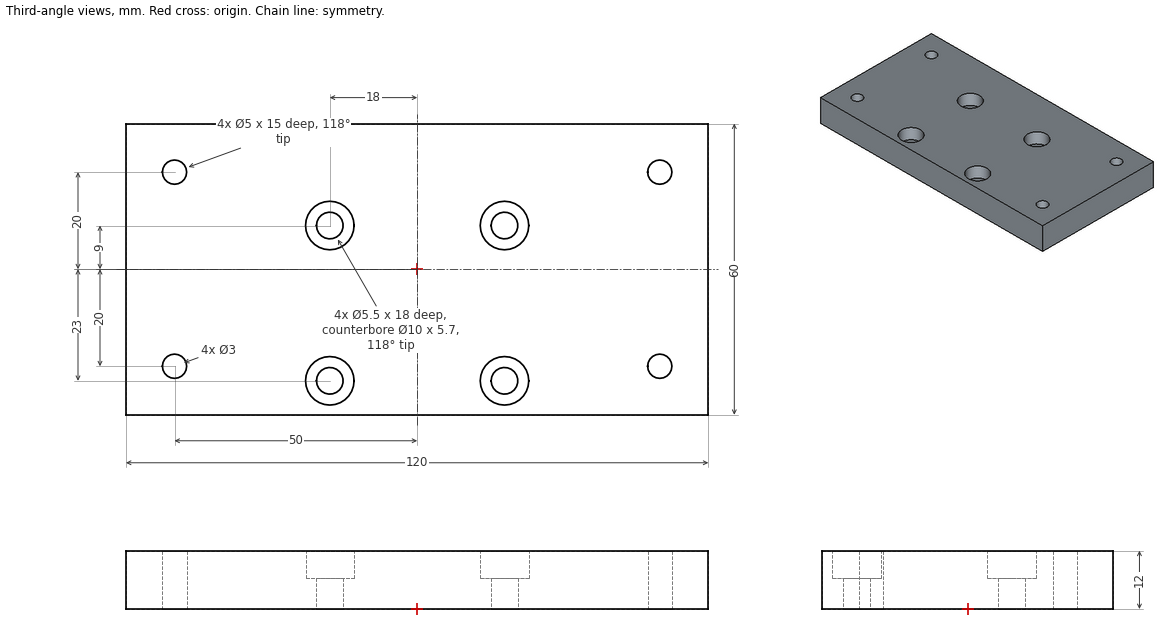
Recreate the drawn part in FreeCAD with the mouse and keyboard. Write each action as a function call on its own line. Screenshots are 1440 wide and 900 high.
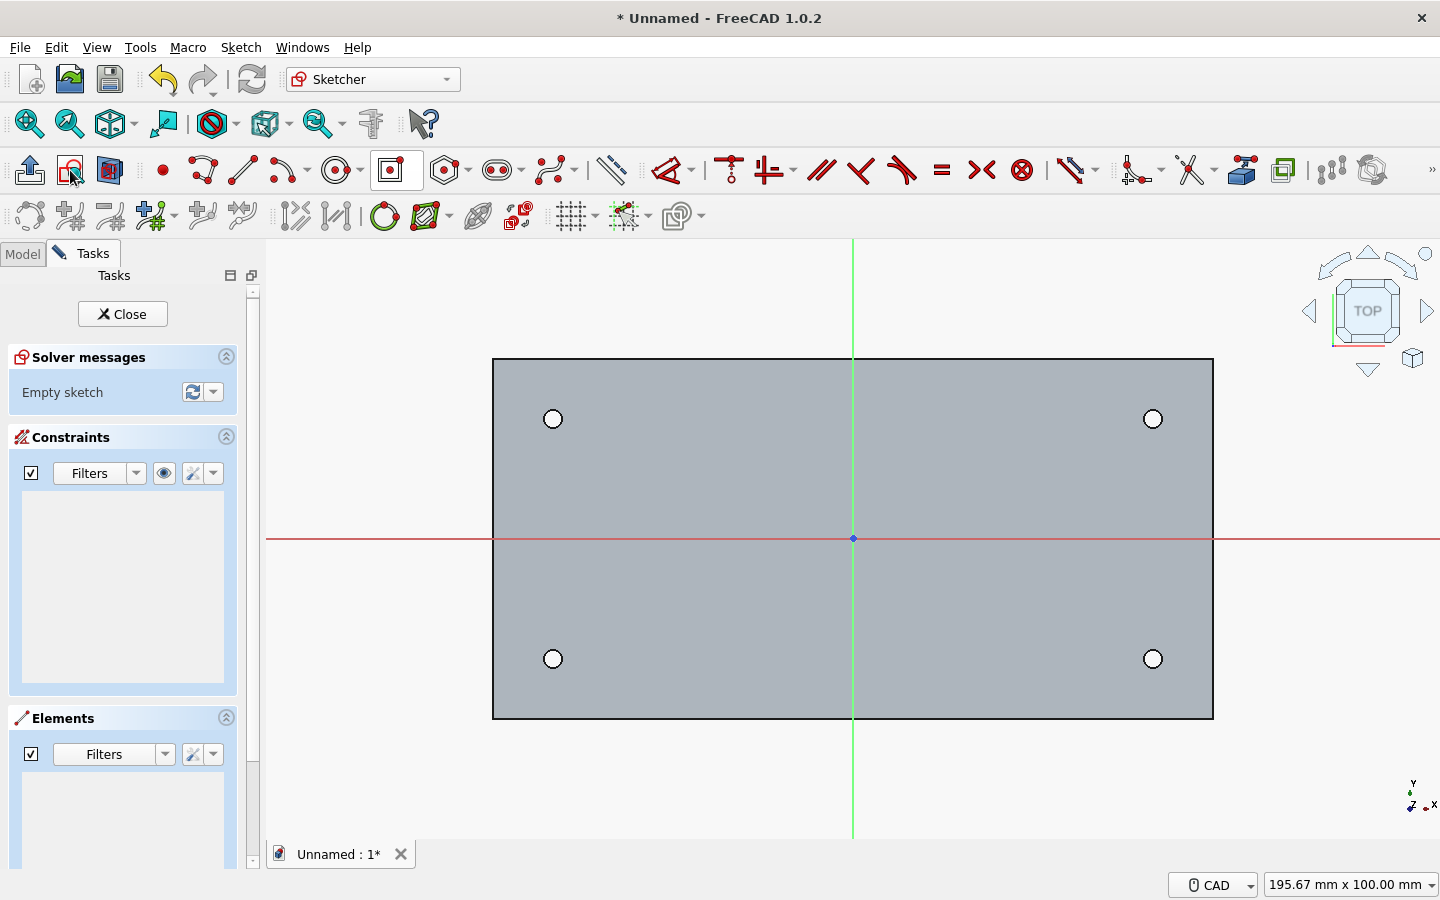
scroll(936, 632, up, 3)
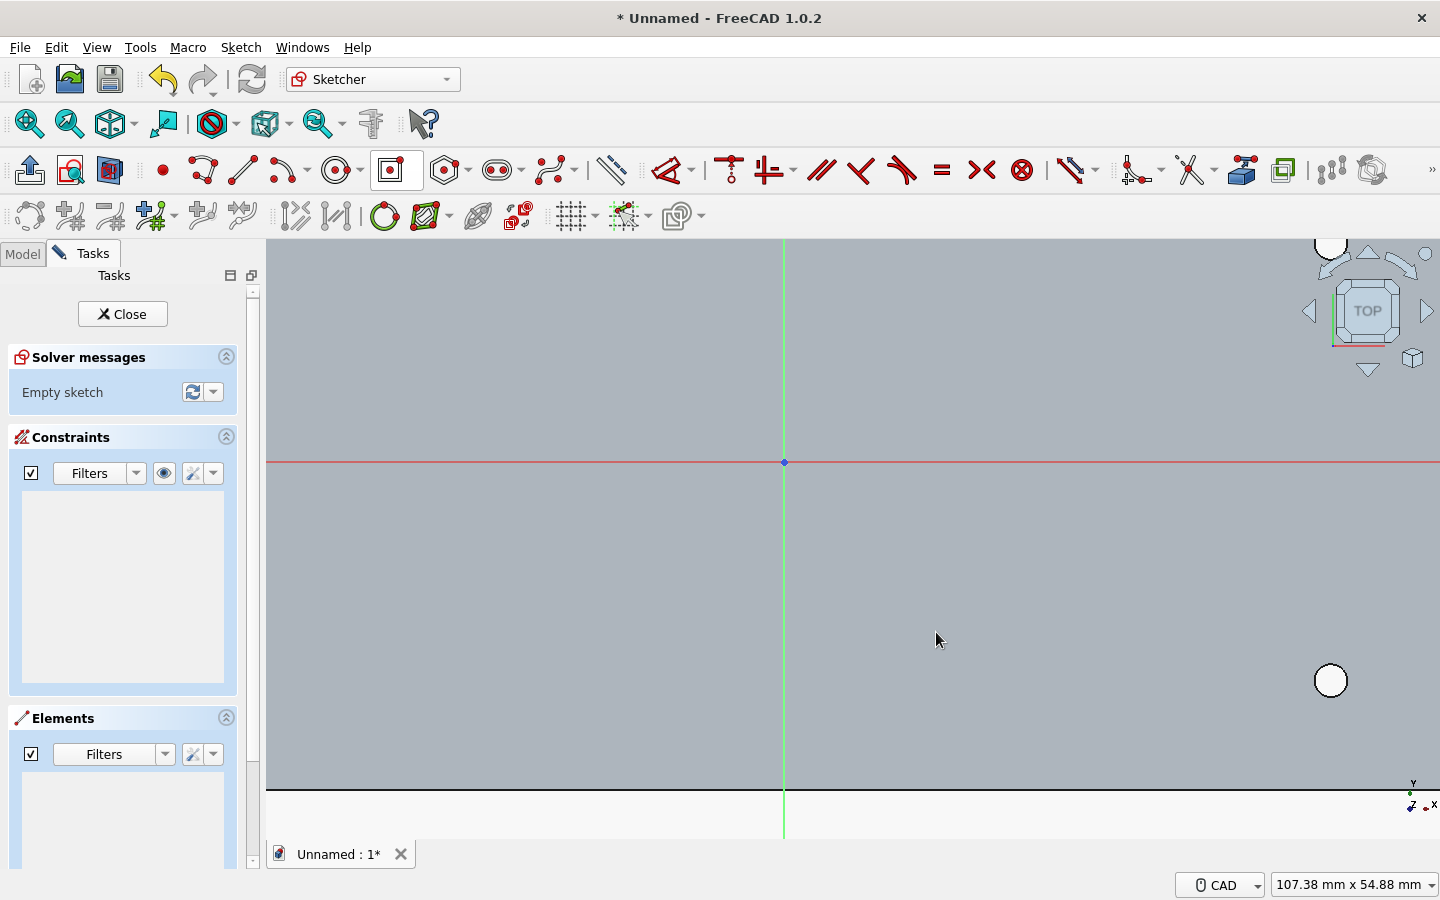
click(336, 170)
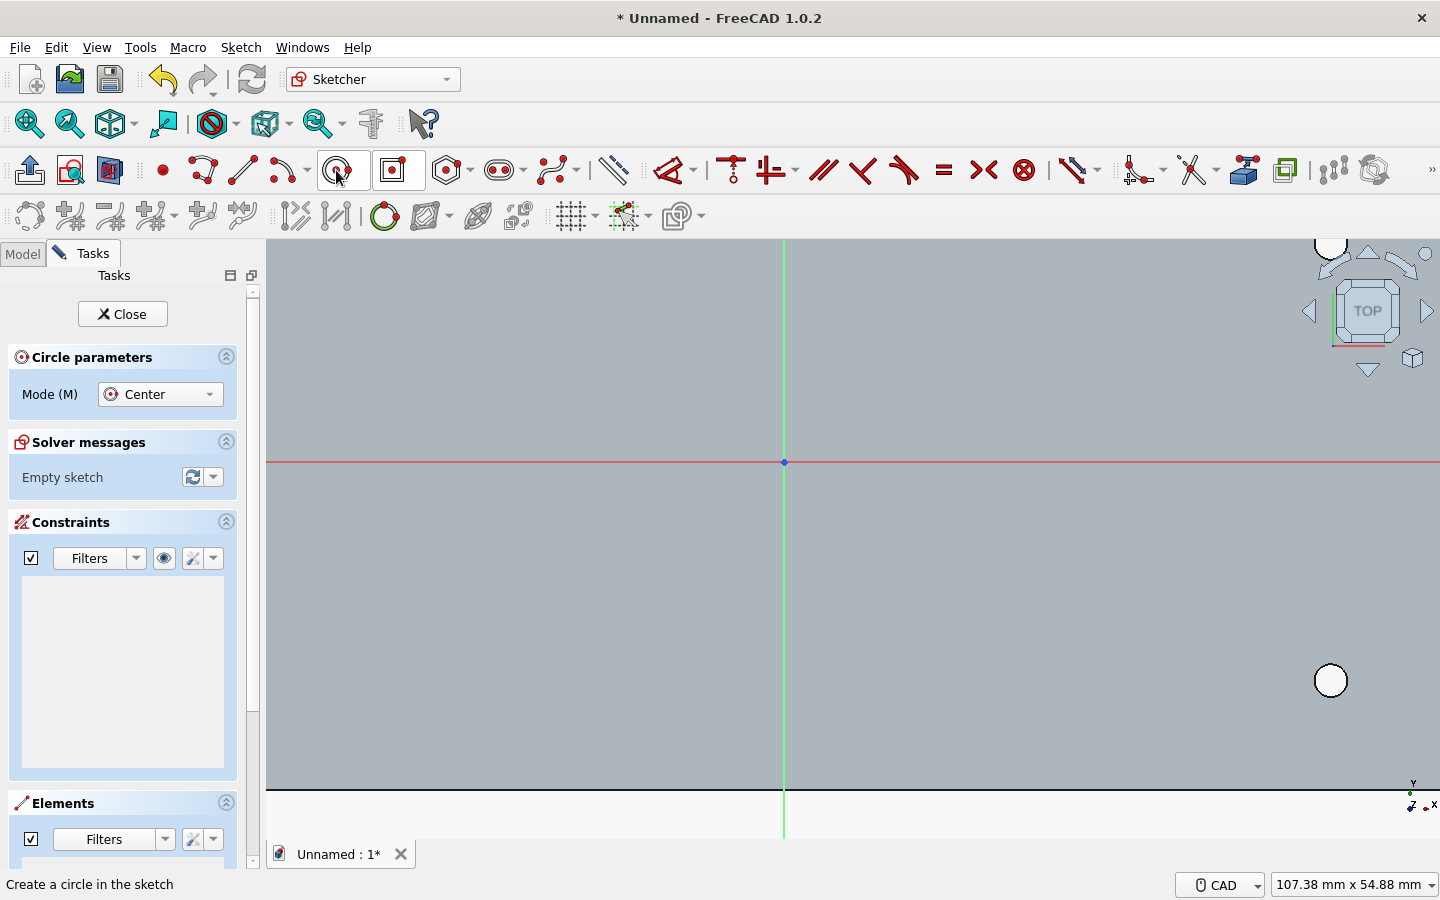
click(588, 364)
click(609, 342)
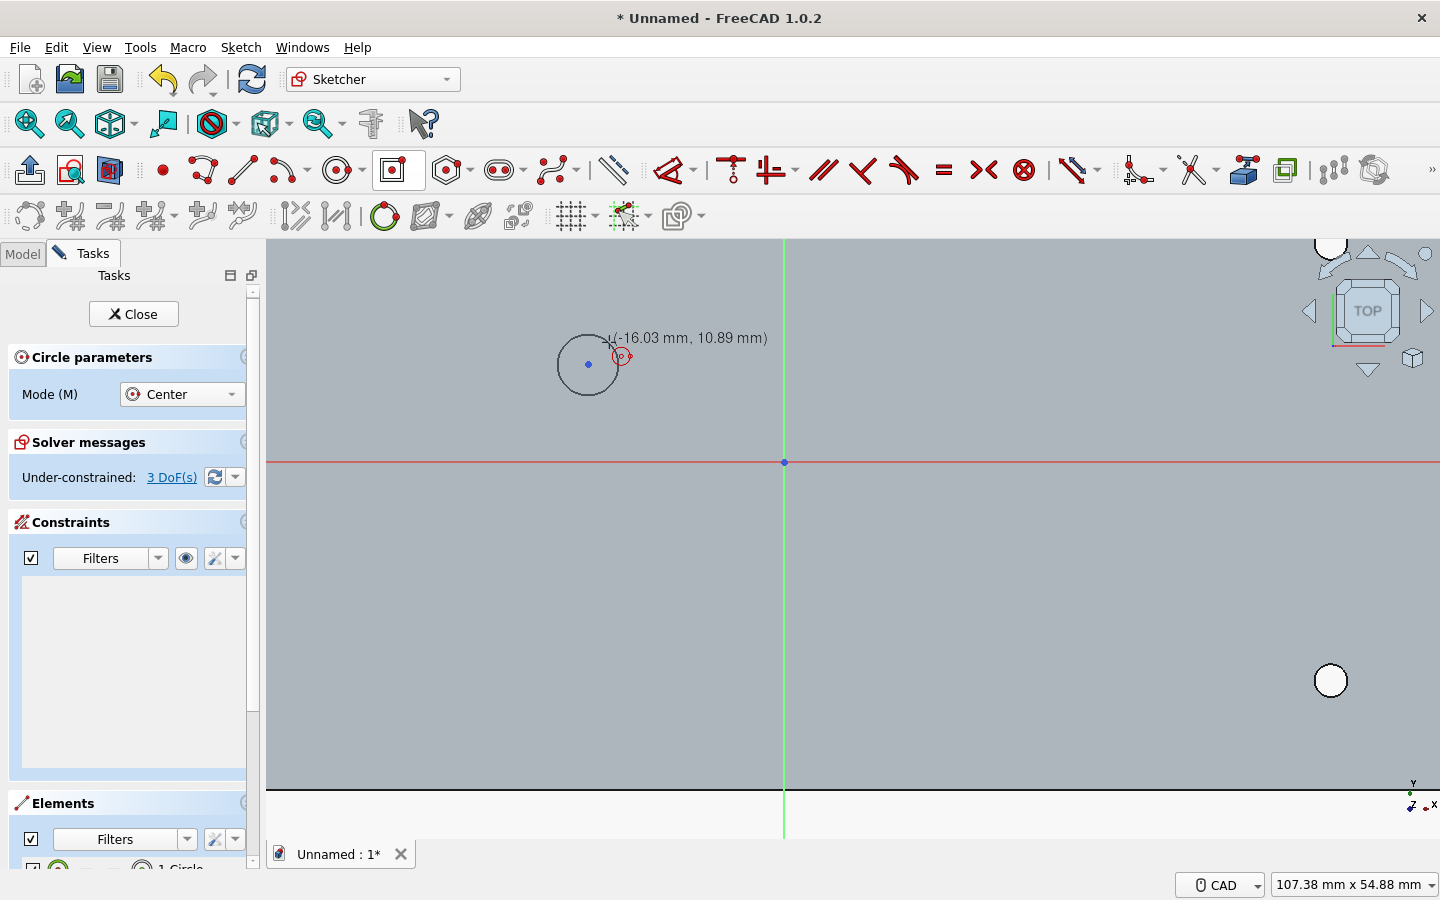
click(981, 364)
click(1002, 342)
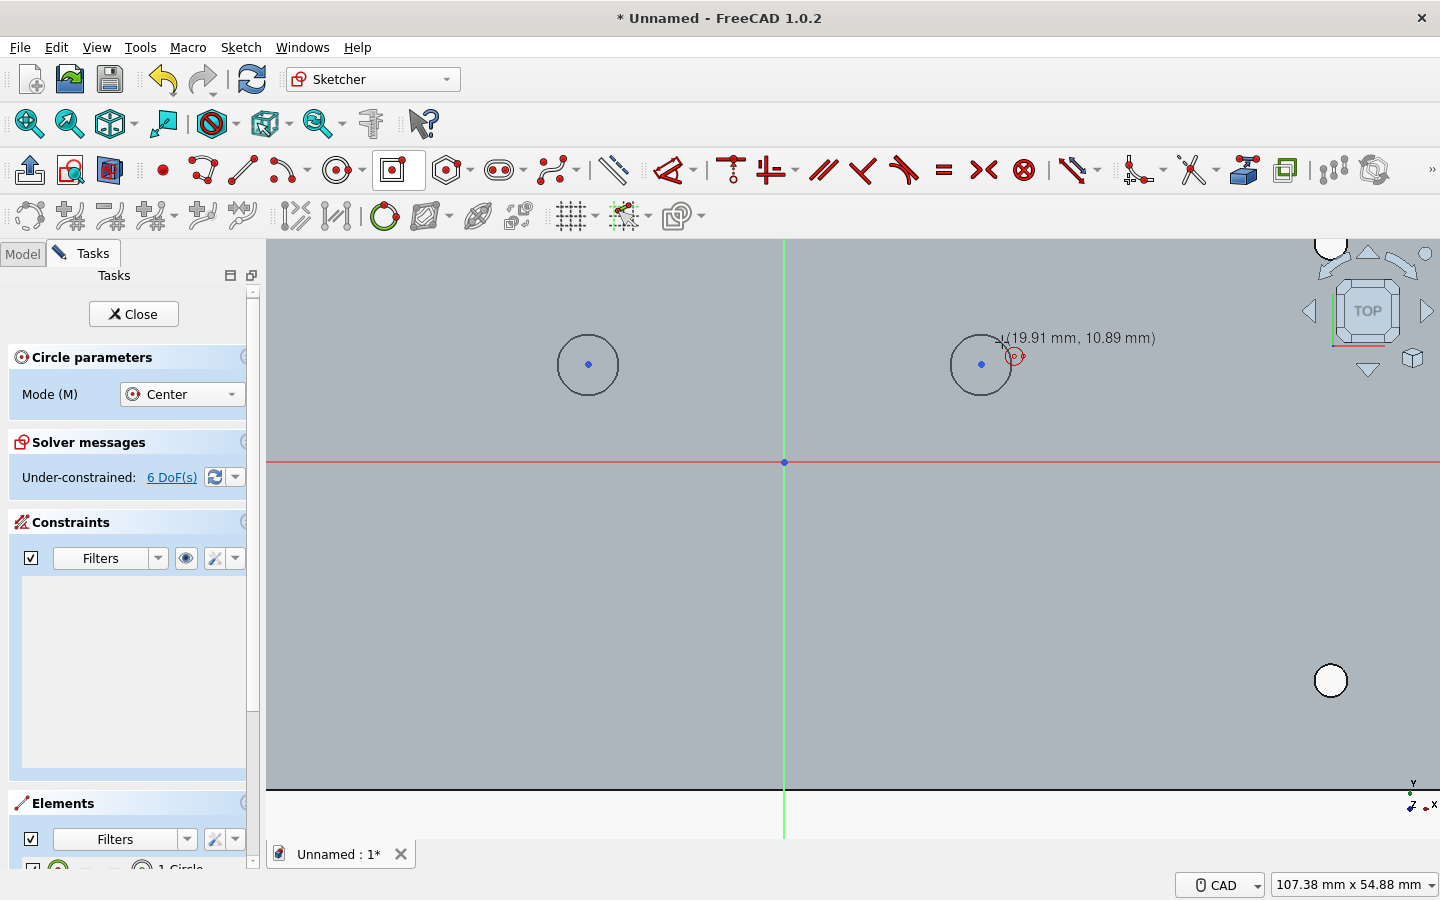
click(588, 713)
click(609, 692)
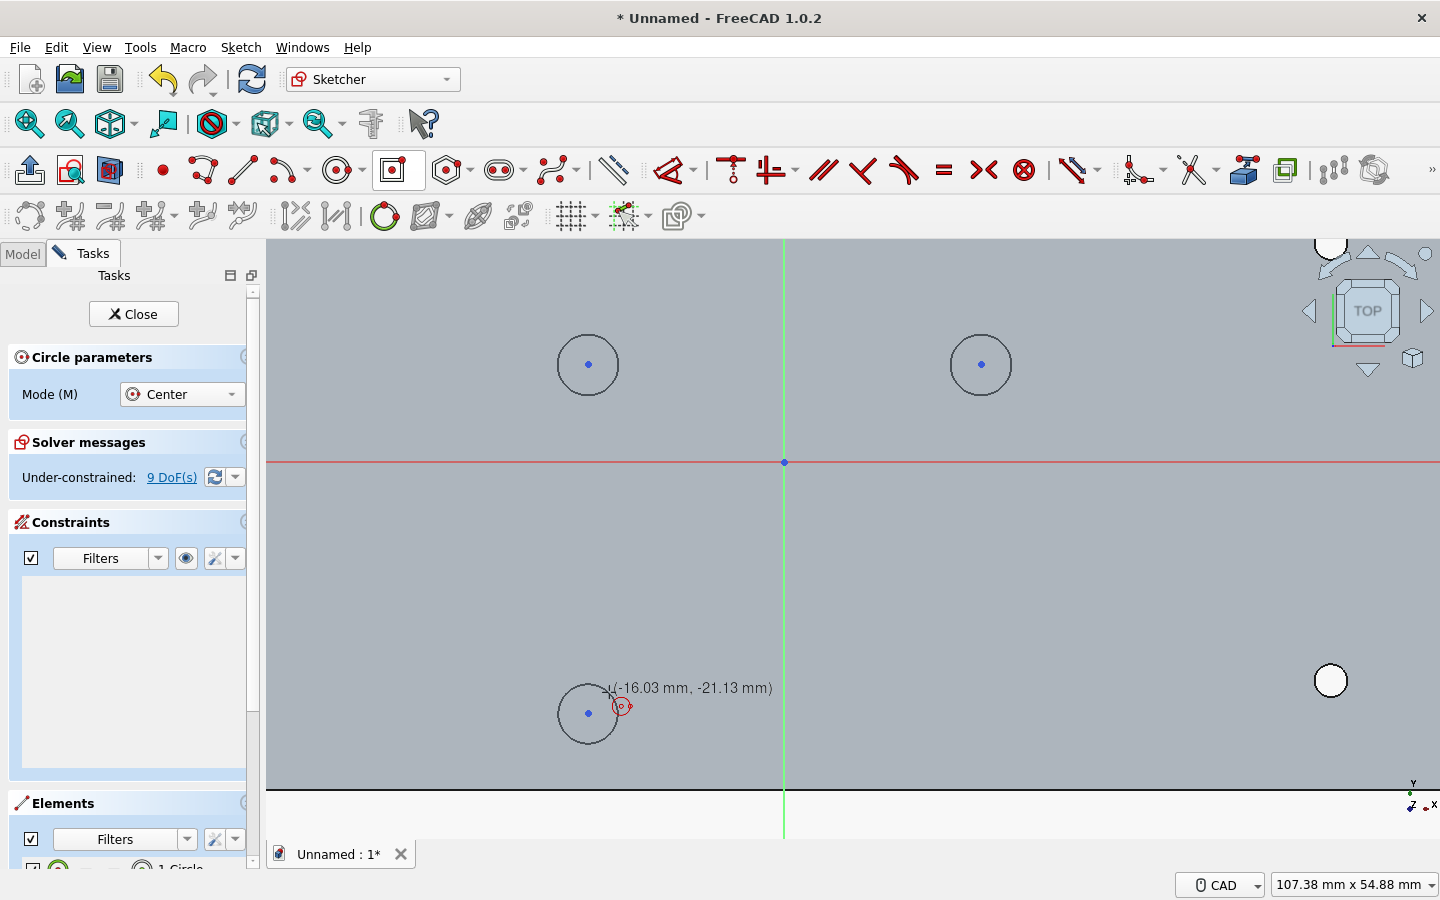
click(981, 713)
click(1002, 692)
key(Escape)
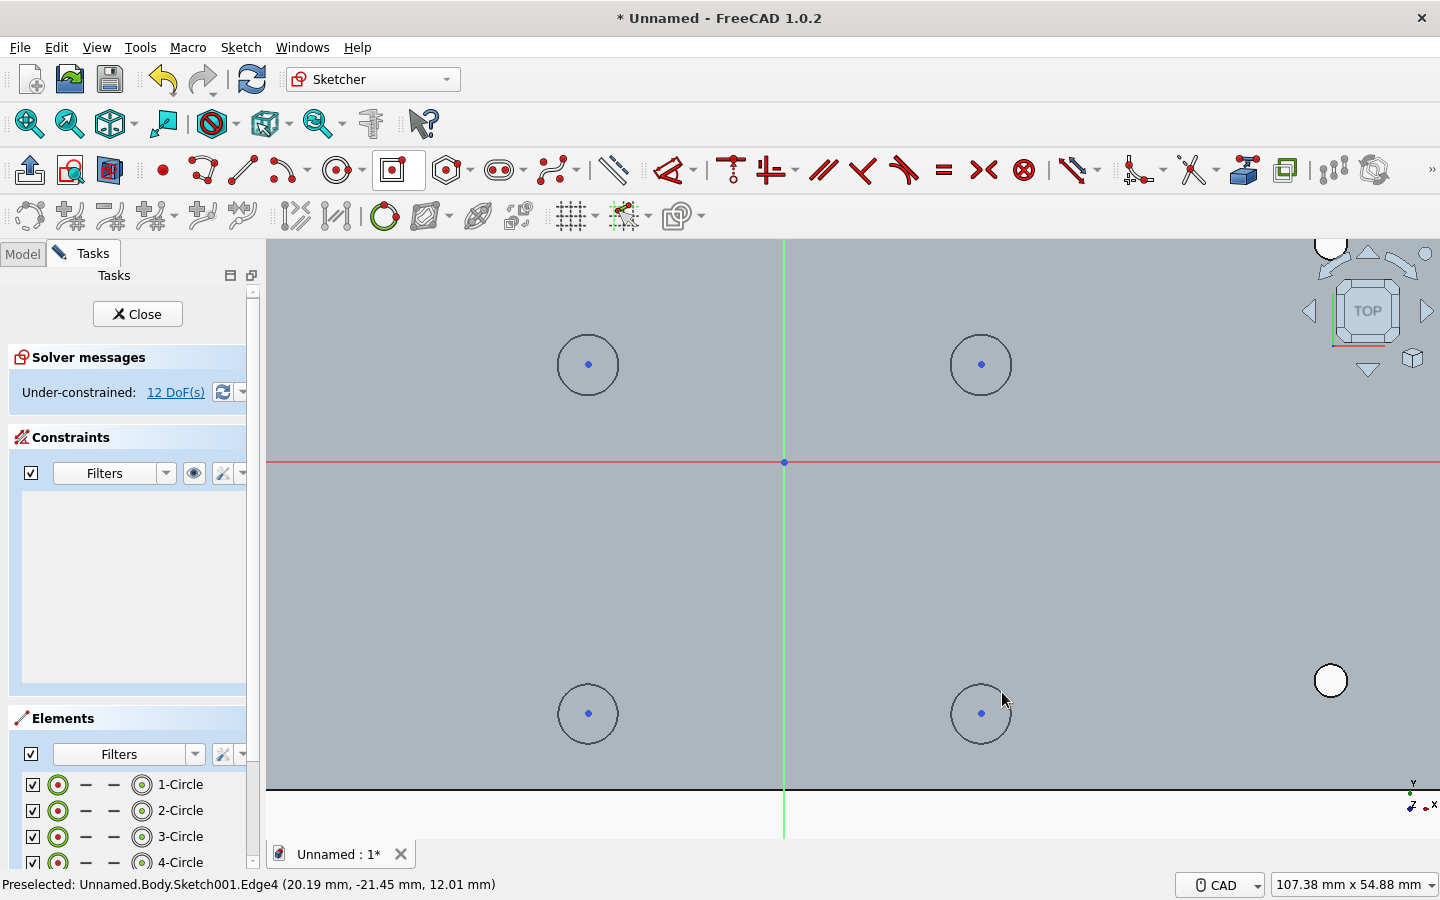
click(609, 343)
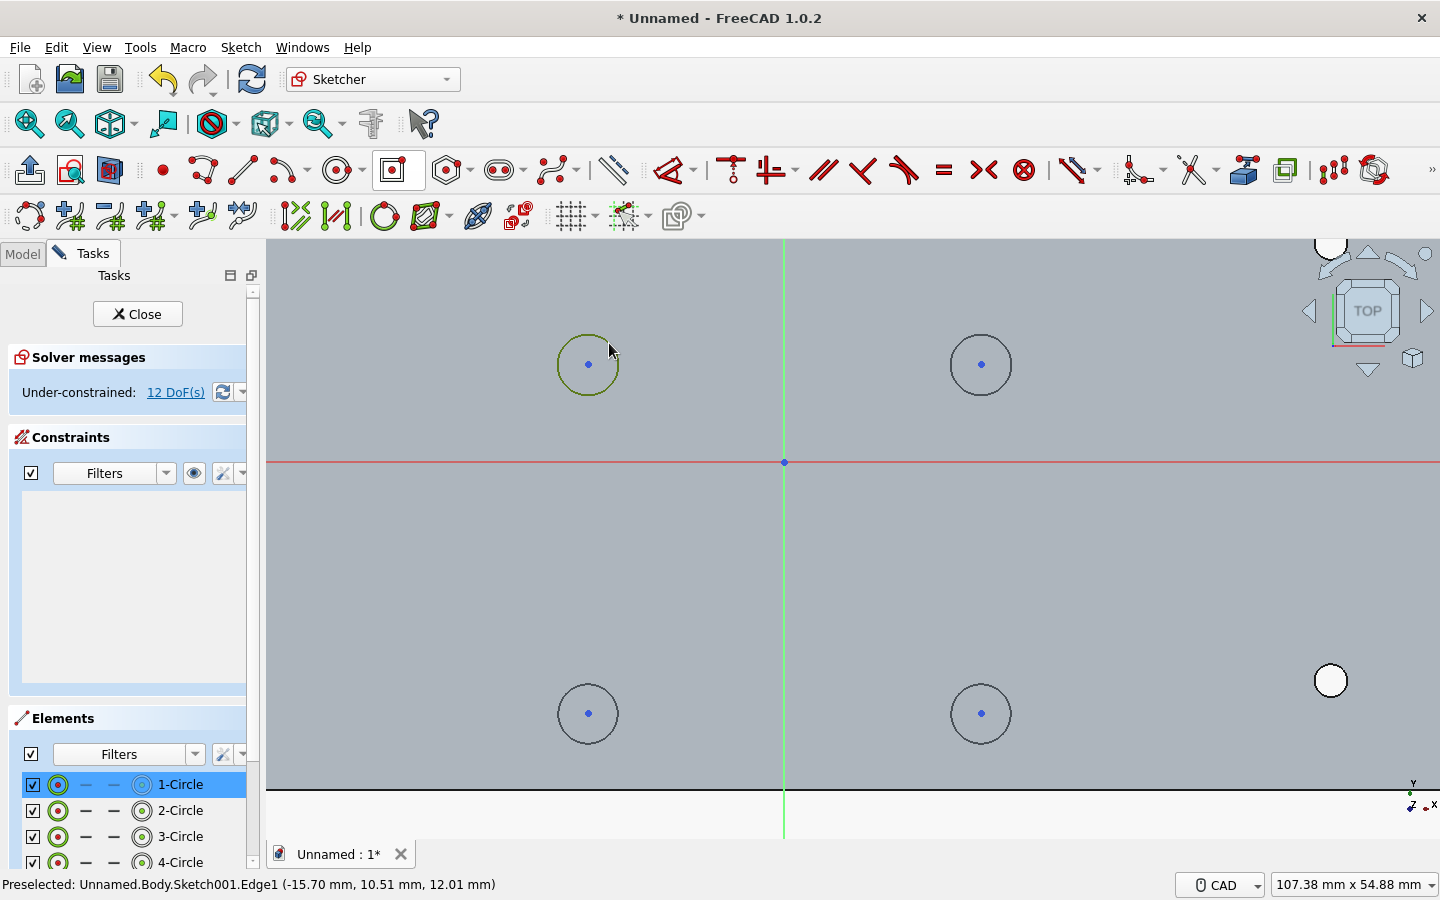
click(1002, 343)